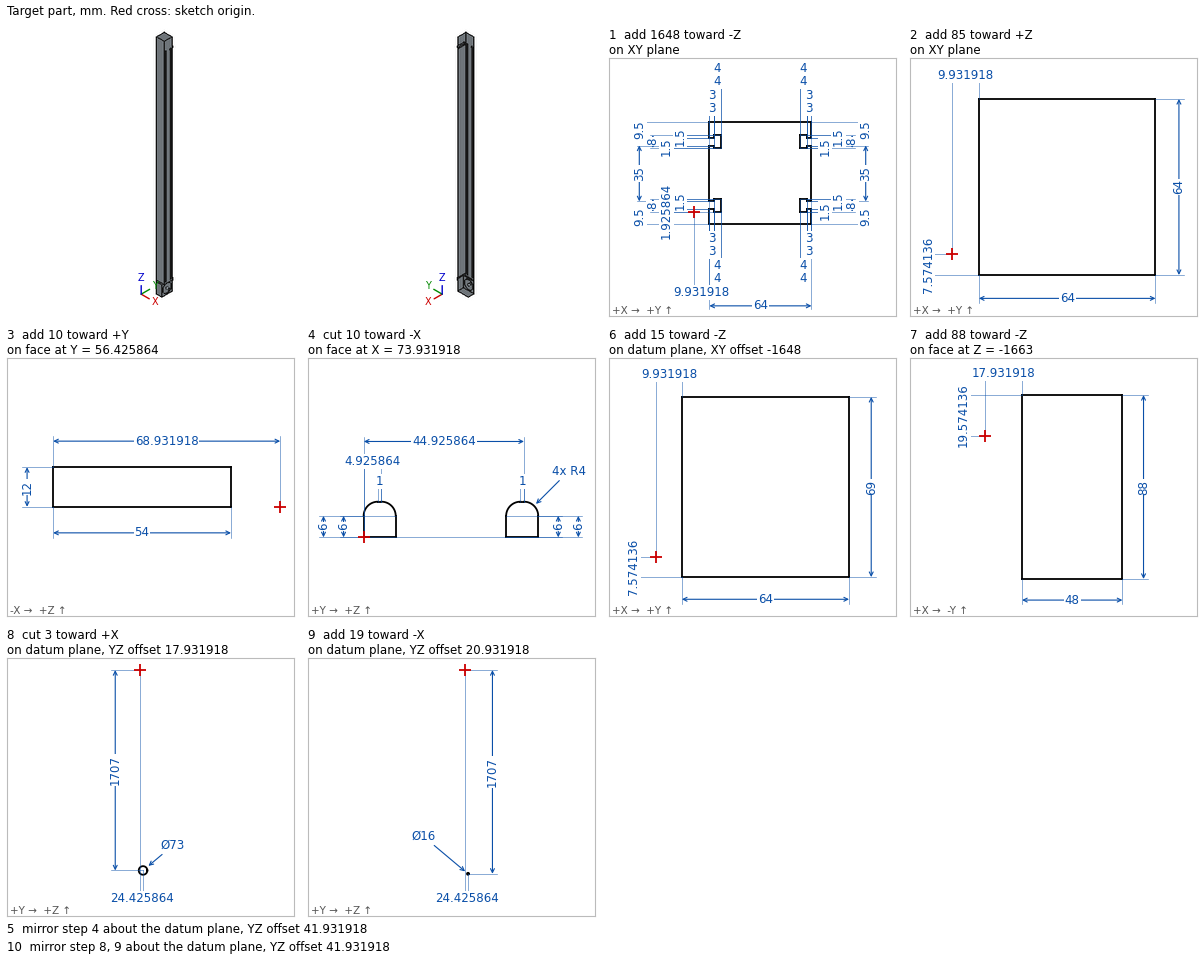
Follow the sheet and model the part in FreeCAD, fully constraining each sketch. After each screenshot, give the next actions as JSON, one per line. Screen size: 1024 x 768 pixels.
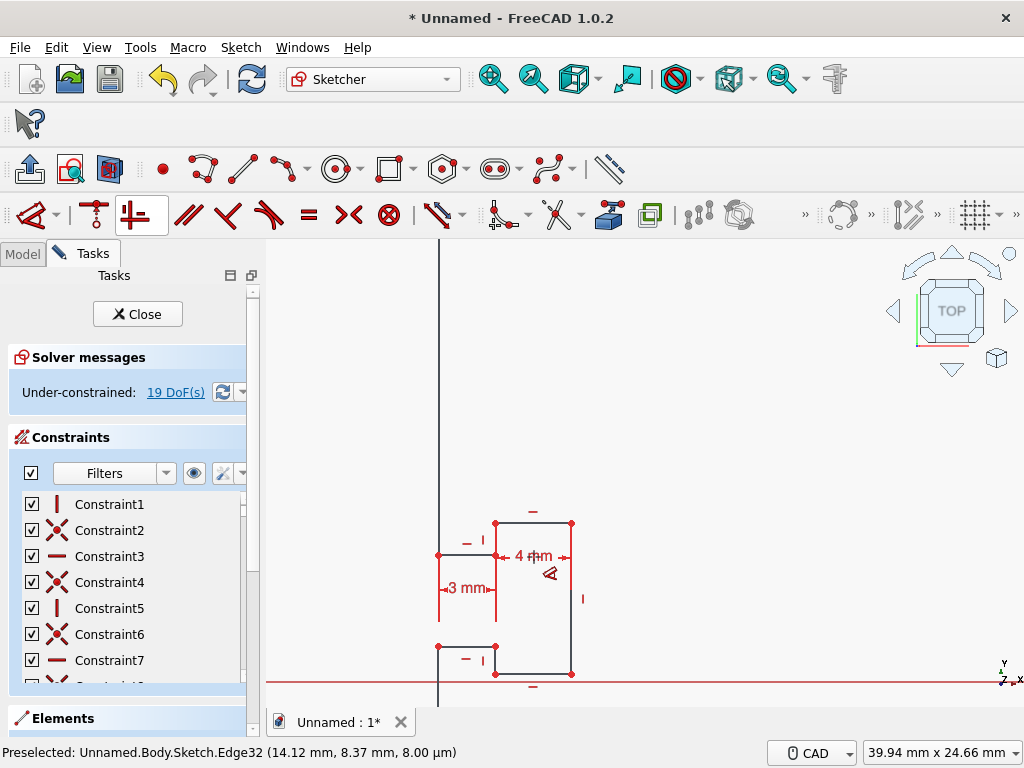
{"action": "scroll", "coordinate": [454, 556], "scroll_direction": "down", "scroll_amount": 7}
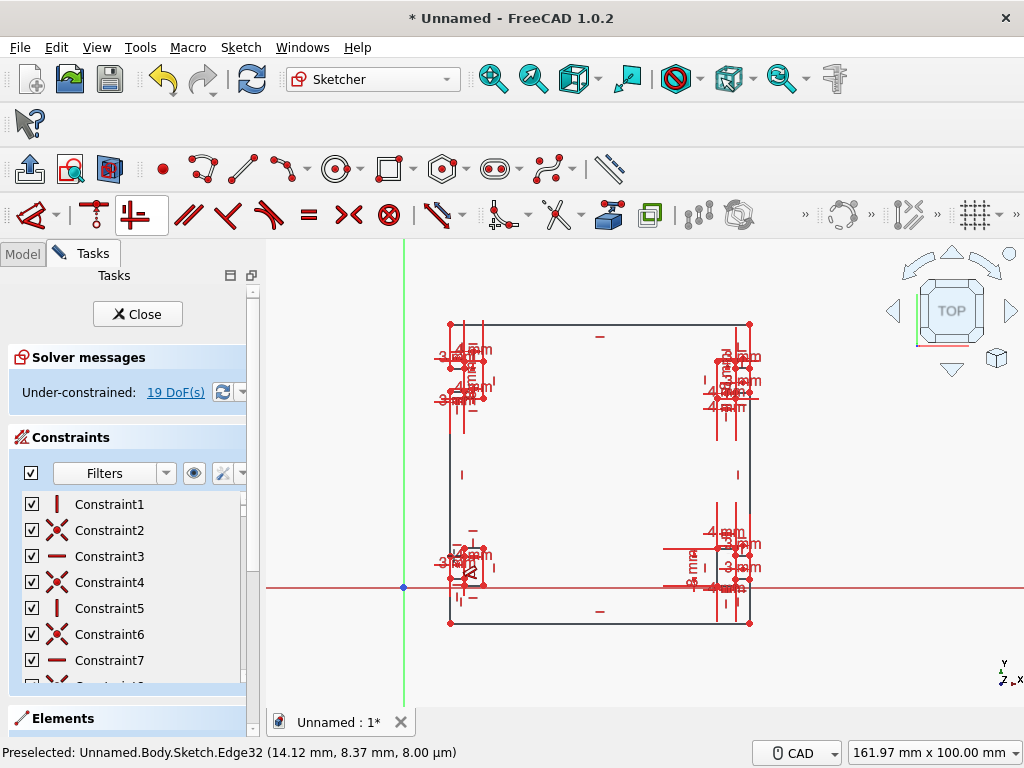
{"action": "scroll", "coordinate": [483, 560], "scroll_direction": "up", "scroll_amount": 2}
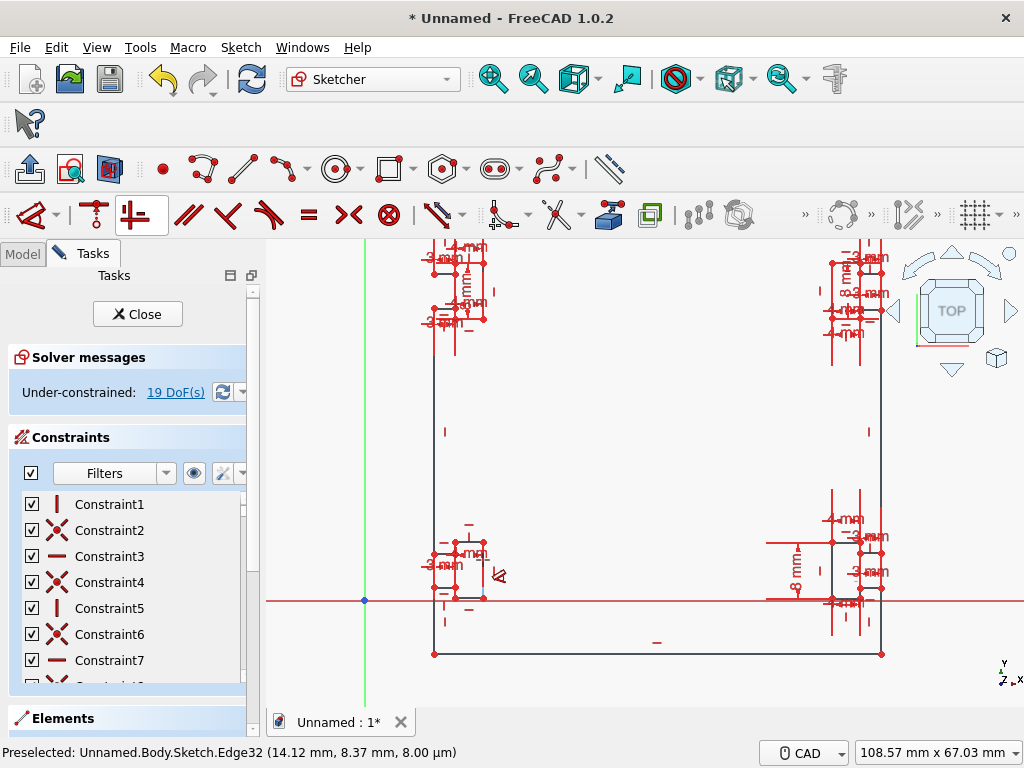
{"action": "left_click", "coordinate": [483, 559]}
{"action": "left_click", "coordinate": [517, 583]}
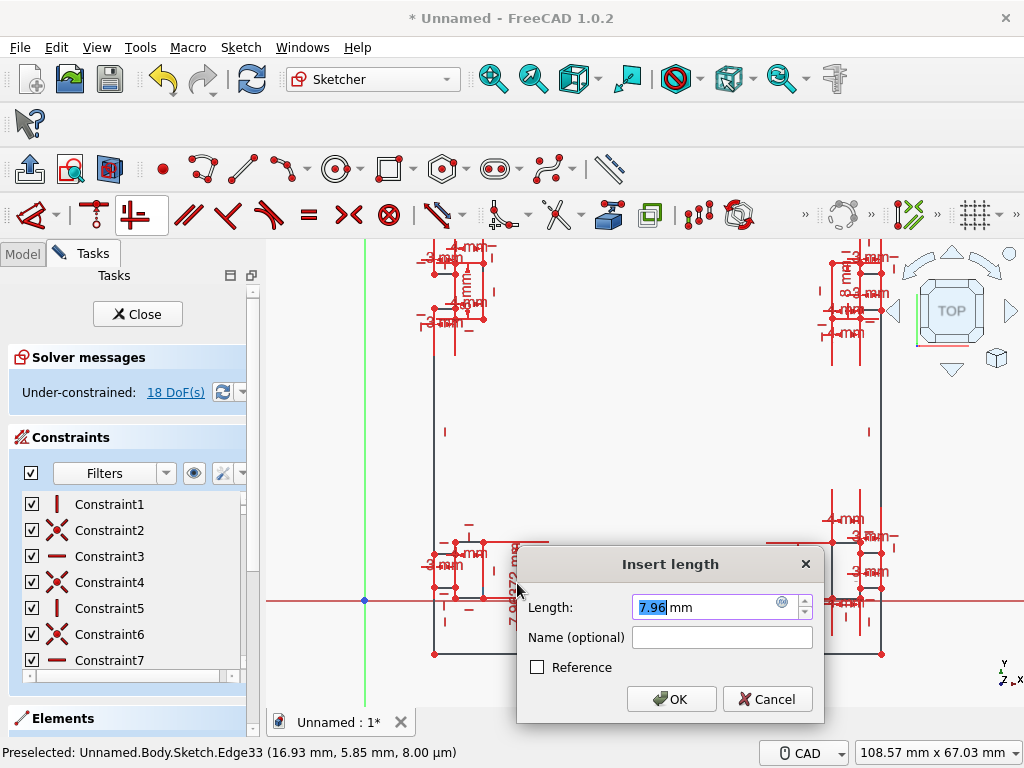
{"action": "type", "text": "8"}
{"action": "key", "text": "Return"}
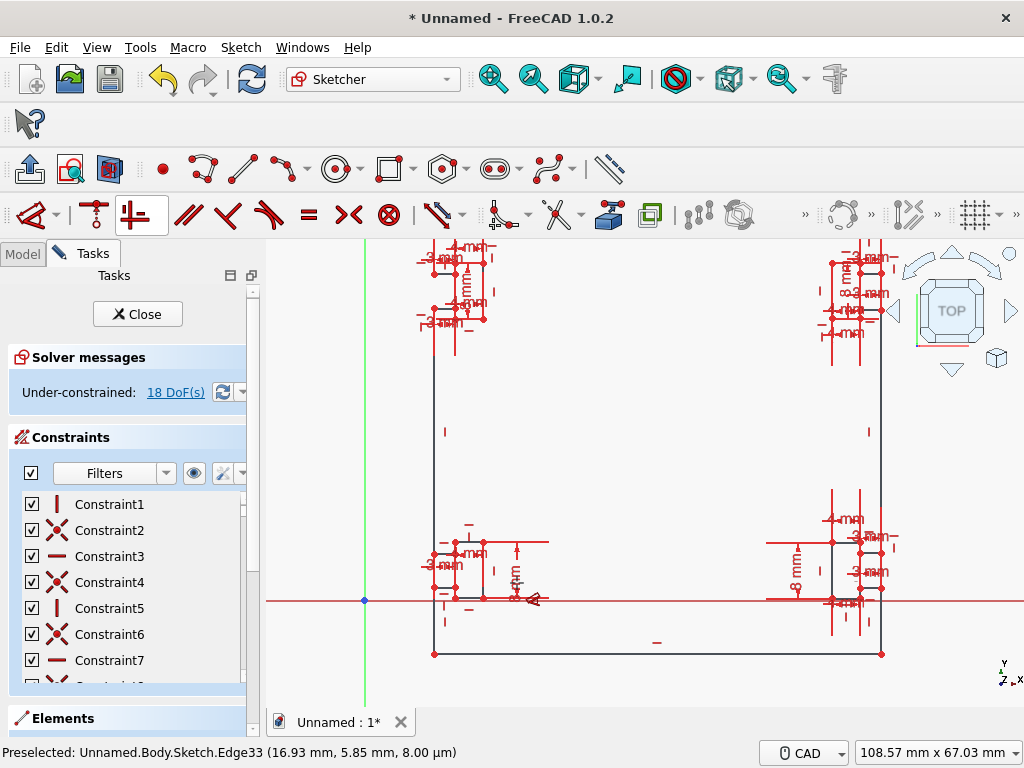
{"action": "scroll", "coordinate": [472, 598], "scroll_direction": "up", "scroll_amount": 2}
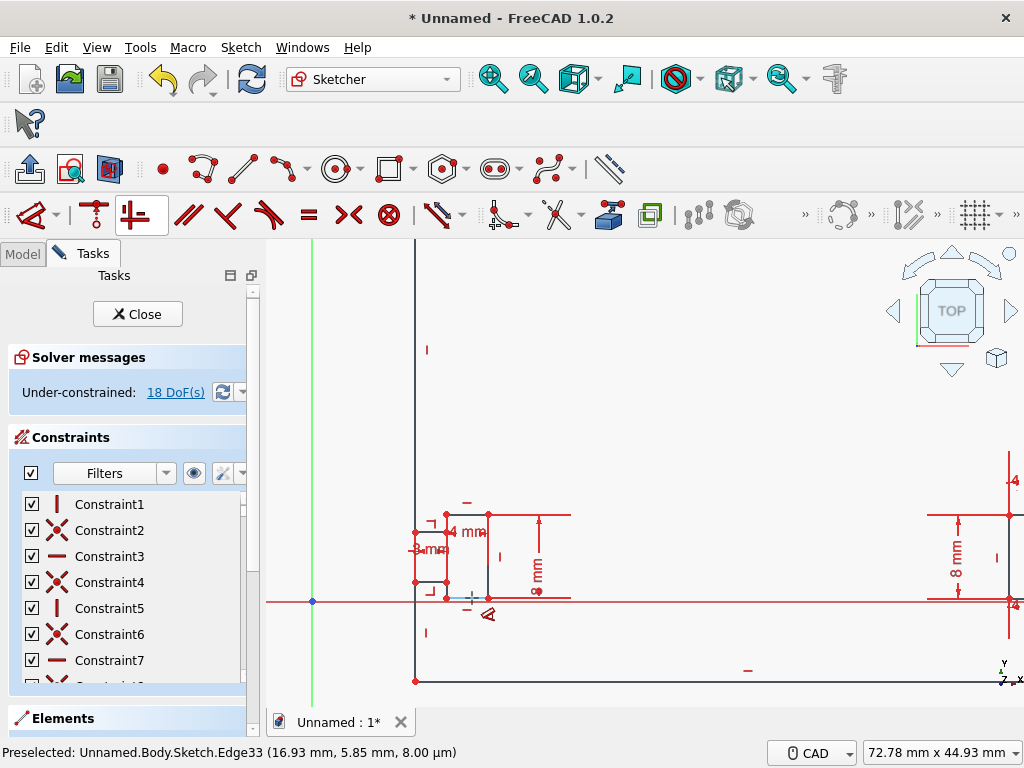
{"action": "left_click", "coordinate": [472, 598]}
{"action": "left_click", "coordinate": [468, 632]}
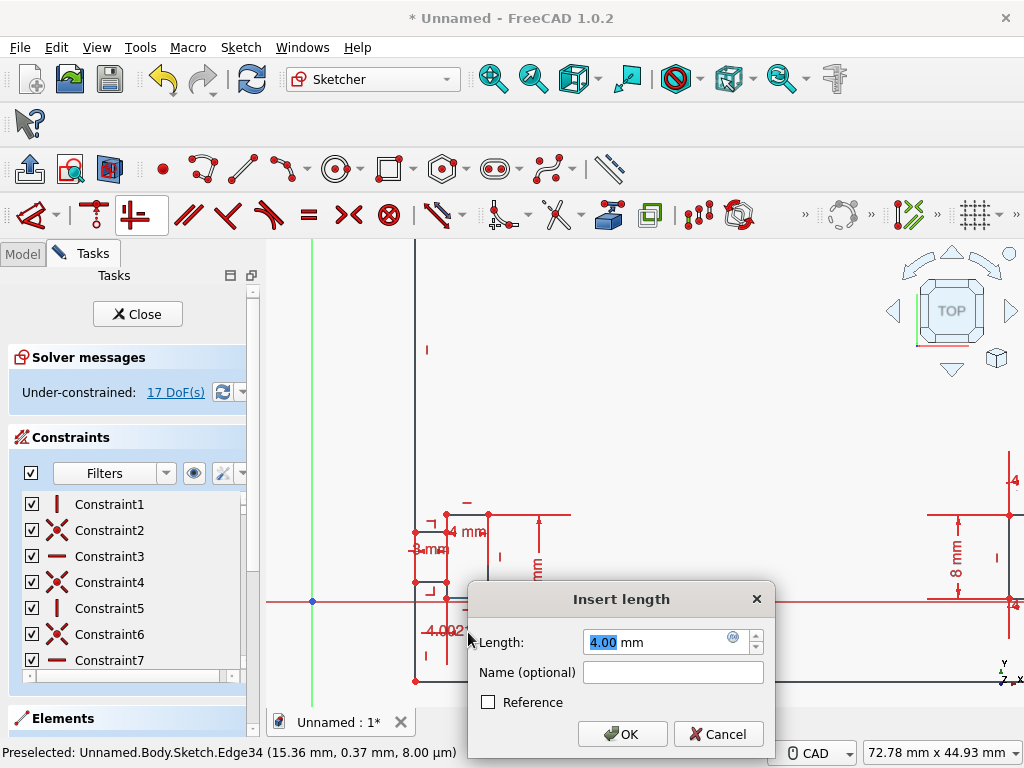
{"action": "type", "text": "4"}
{"action": "key", "text": "Return"}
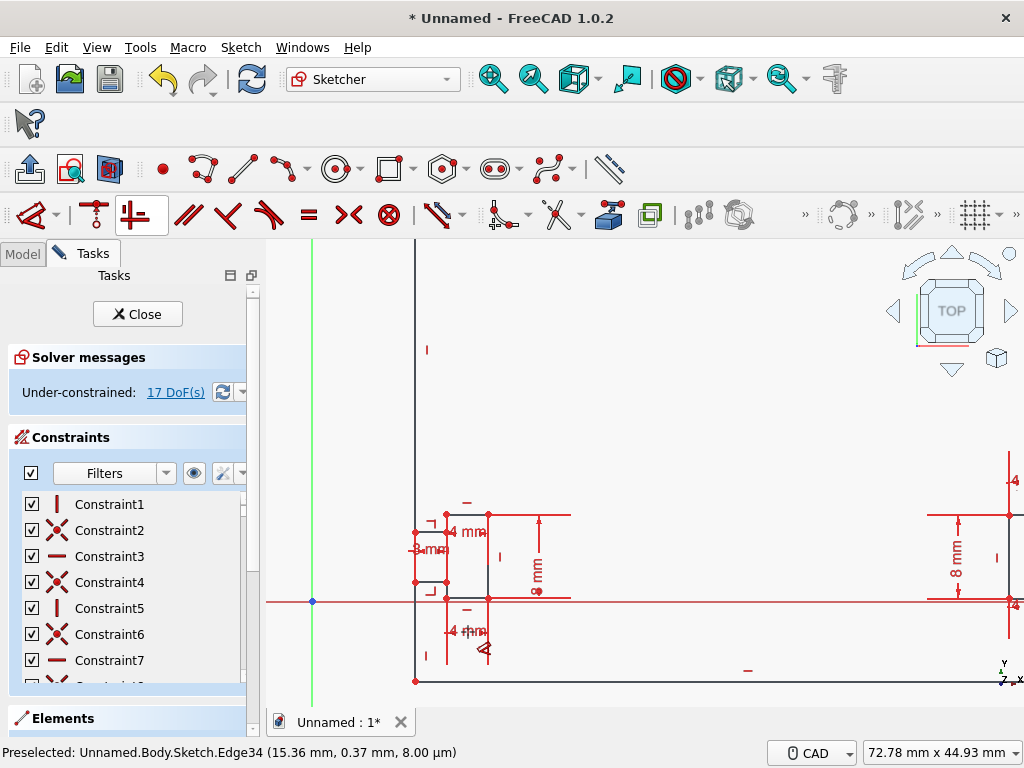
{"action": "scroll", "coordinate": [437, 582], "scroll_direction": "up", "scroll_amount": 2}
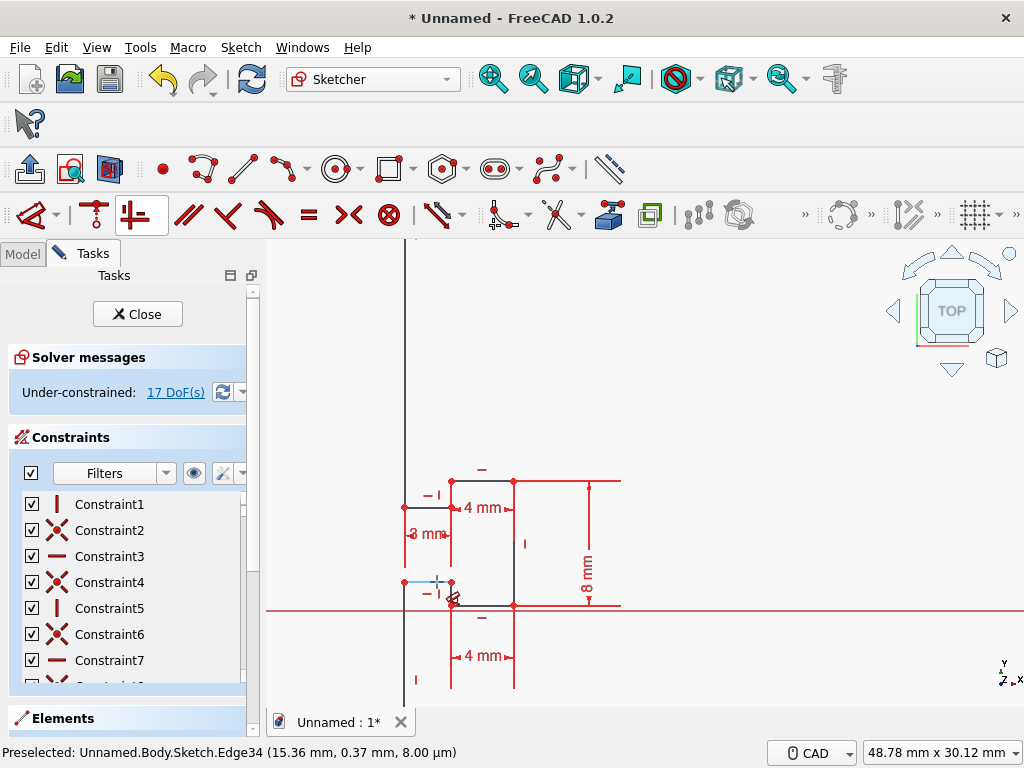
{"action": "left_click", "coordinate": [437, 582]}
{"action": "left_click", "coordinate": [428, 476]}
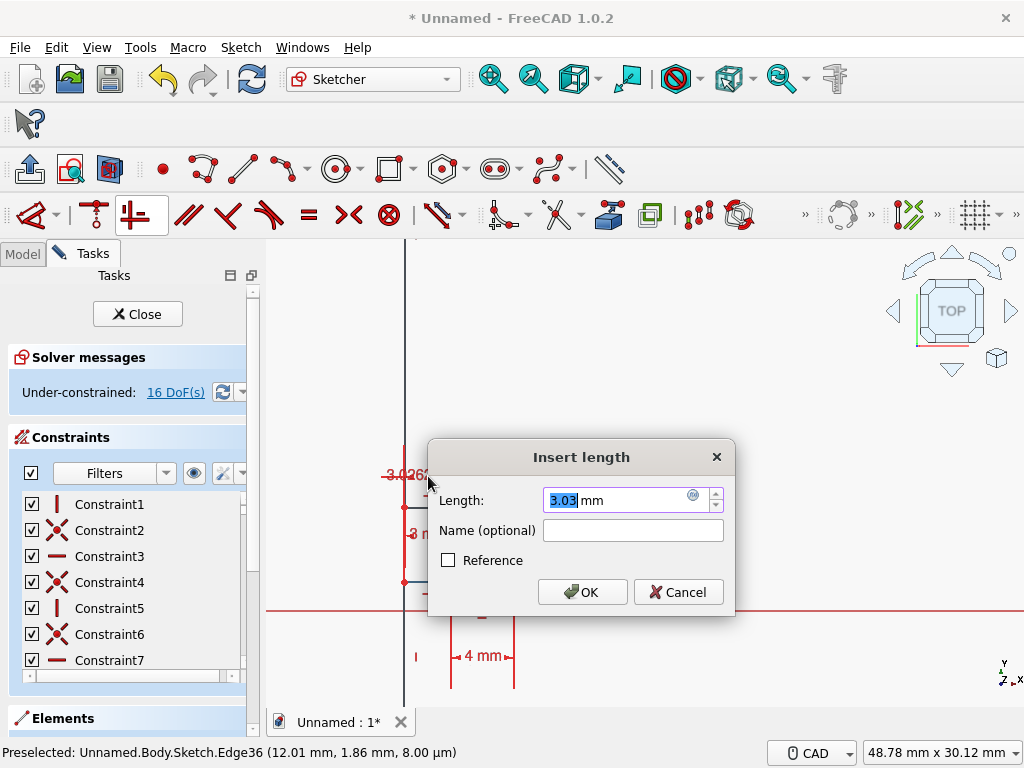
{"action": "type", "text": "3"}
{"action": "key", "text": "Return"}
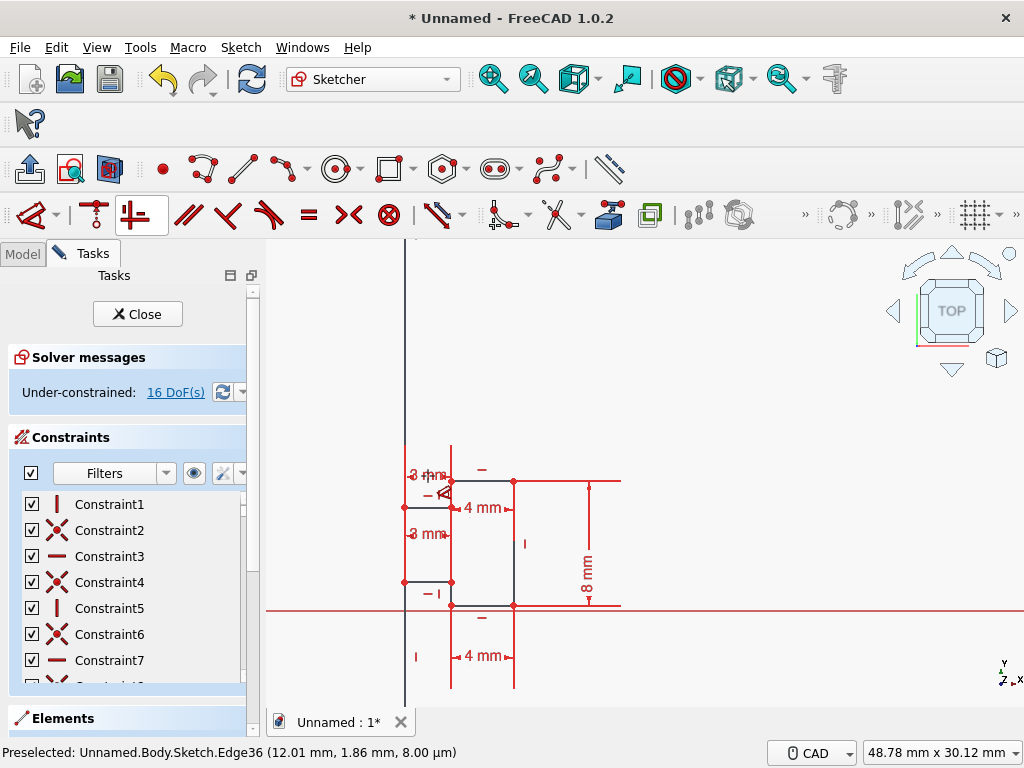
{"action": "scroll", "coordinate": [469, 577], "scroll_direction": "down", "scroll_amount": 6}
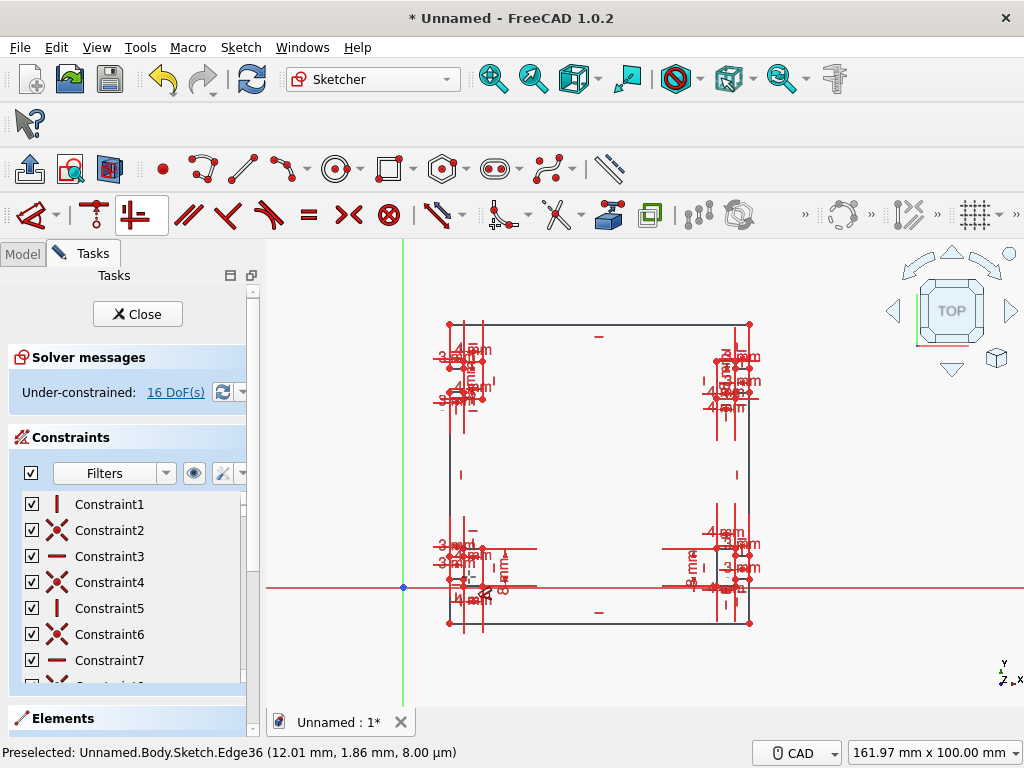
{"action": "left_click", "coordinate": [540, 624]}
{"action": "left_click", "coordinate": [600, 658]}